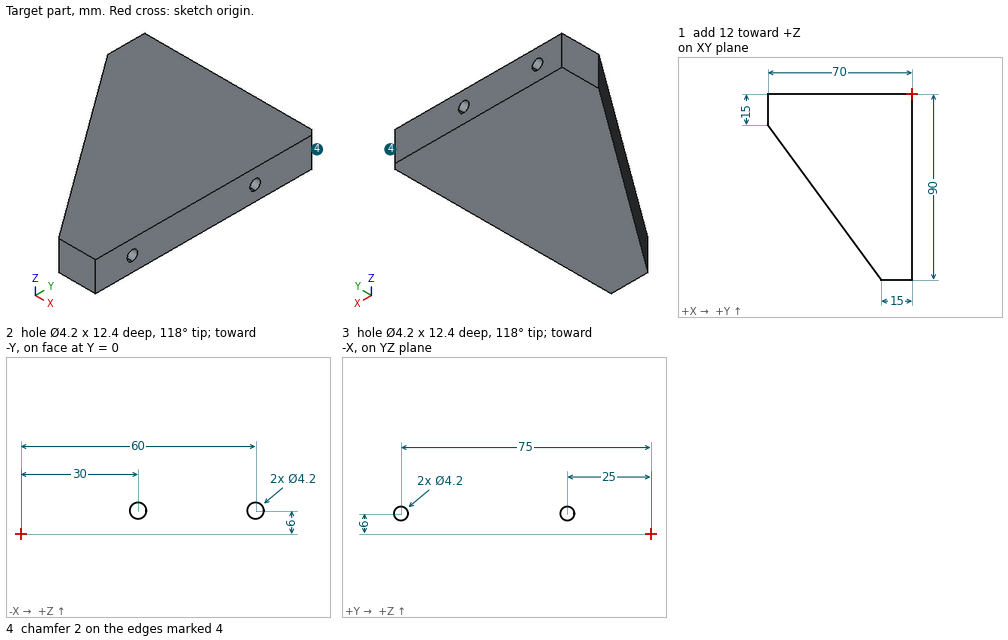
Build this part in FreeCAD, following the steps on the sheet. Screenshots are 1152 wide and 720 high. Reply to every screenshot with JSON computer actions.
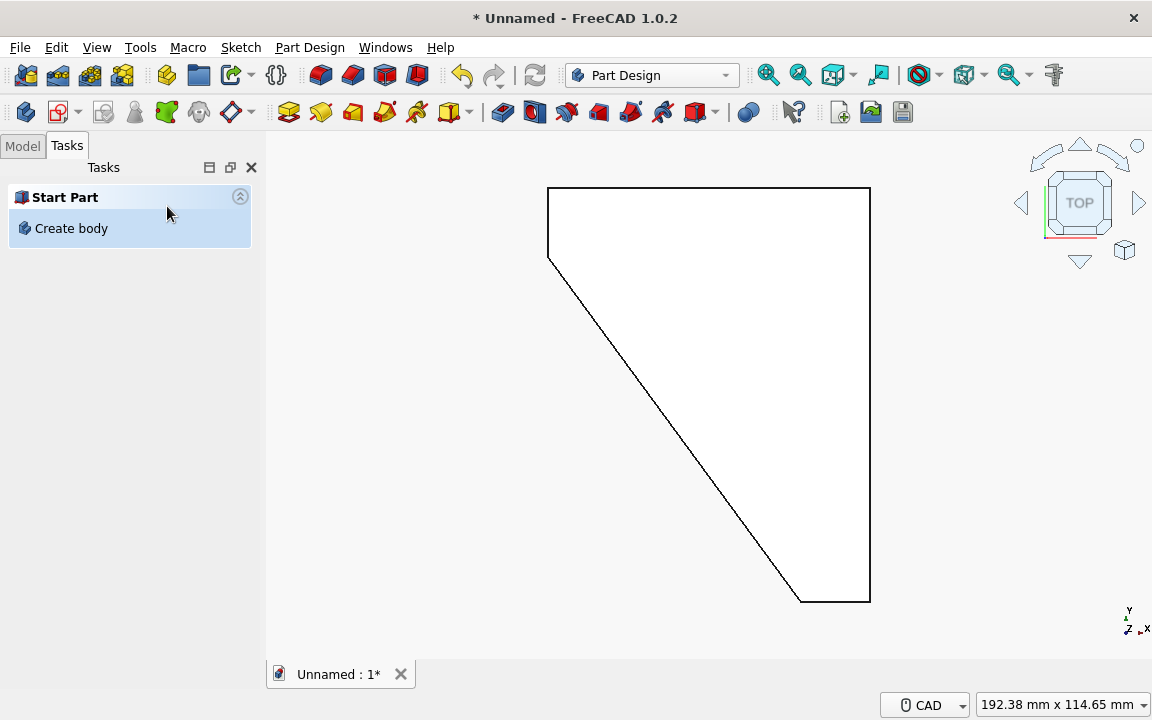
{"action": "key", "text": "1"}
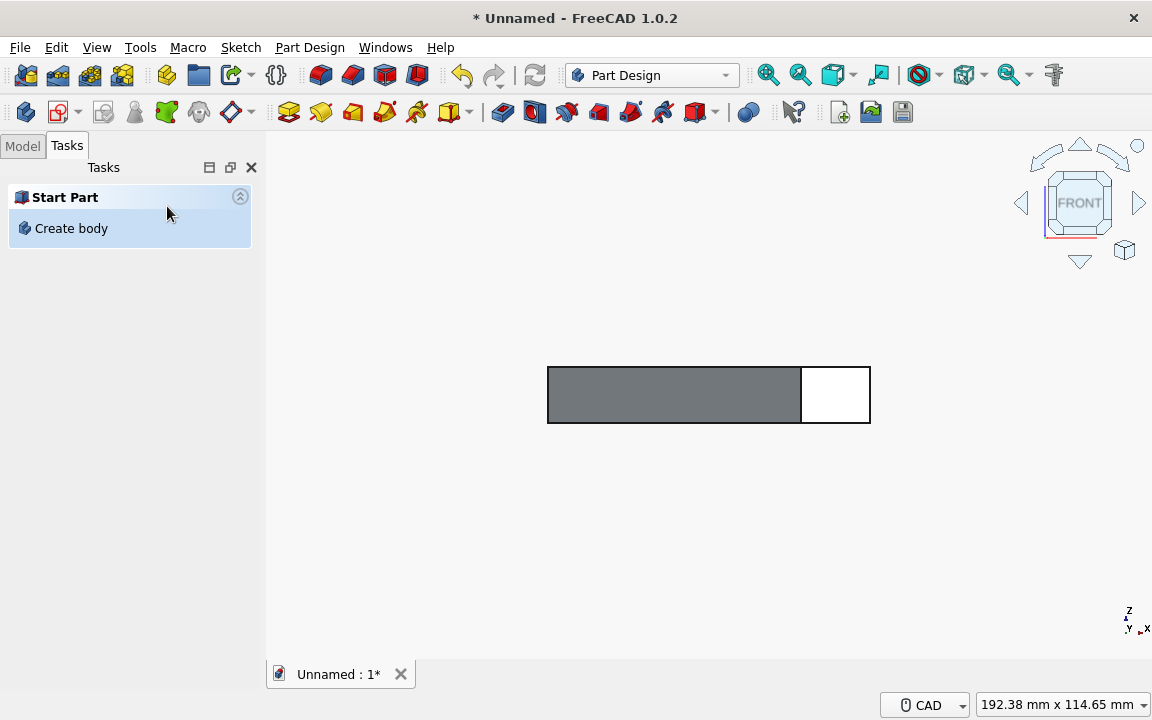
{"action": "left_click", "coordinate": [770, 76]}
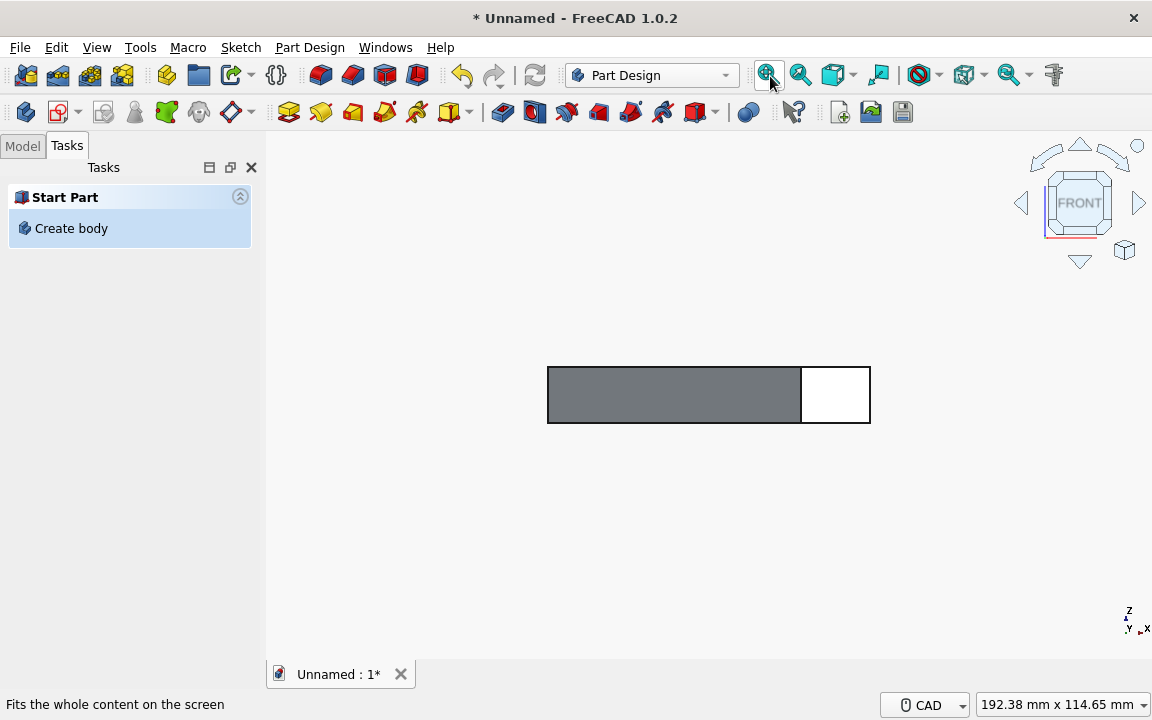
{"action": "key", "text": "3"}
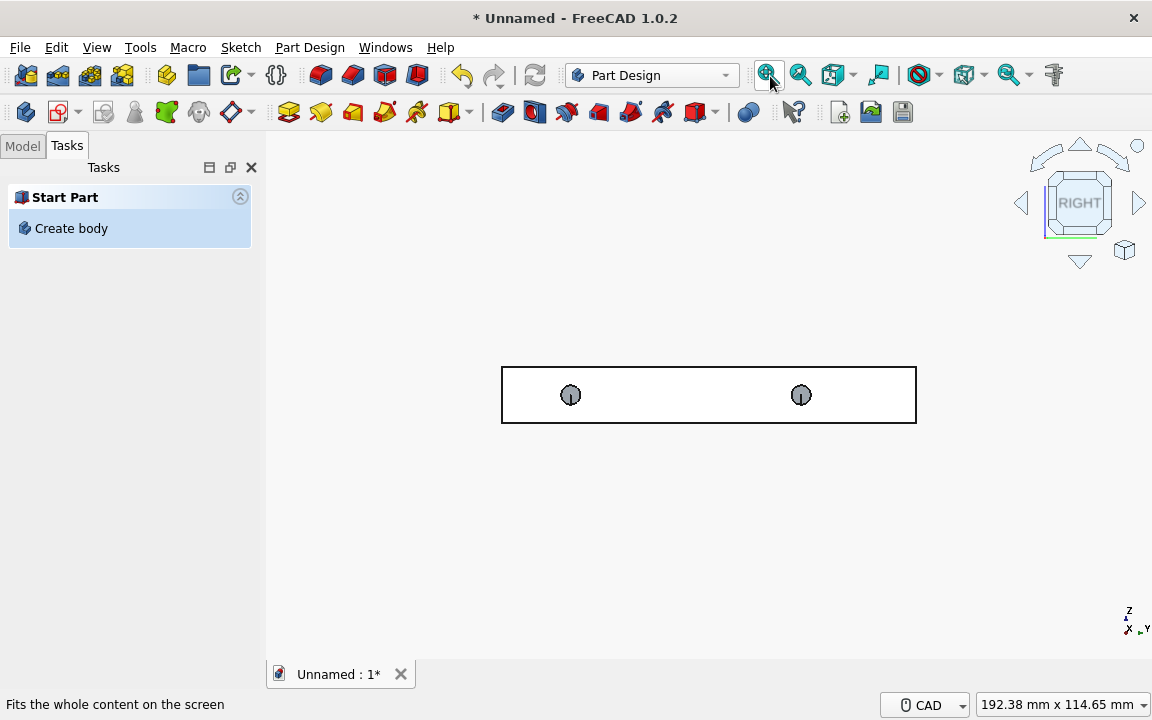
{"action": "left_click", "coordinate": [916, 394]}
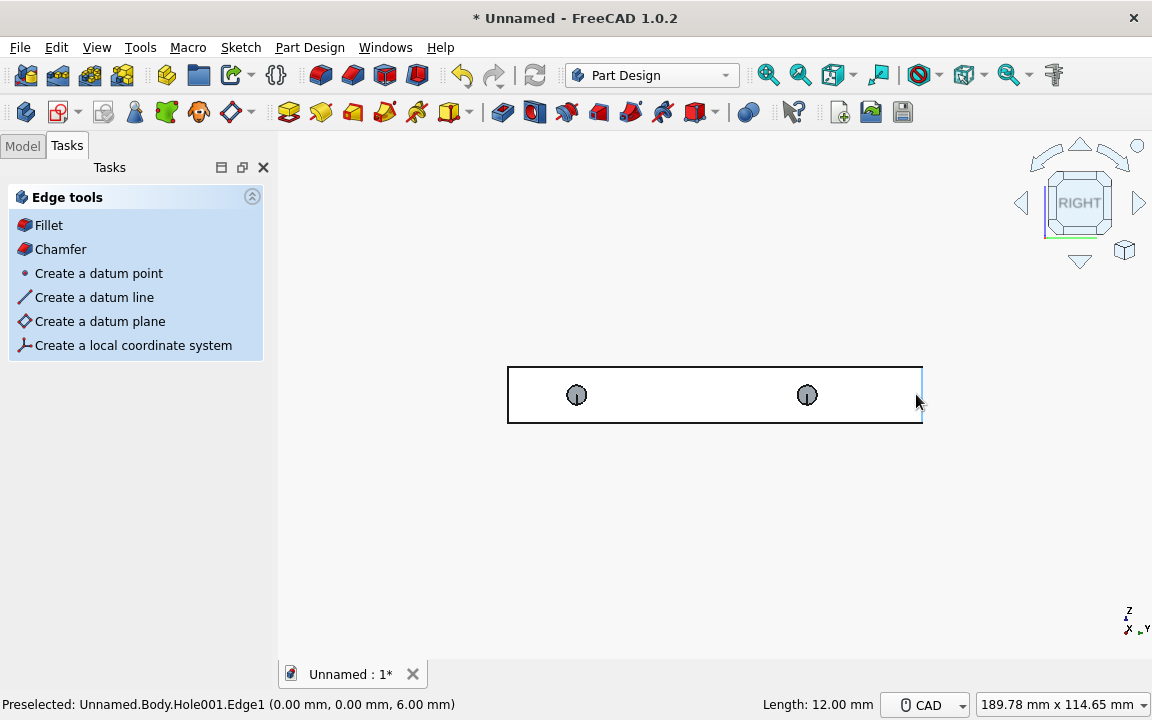
{"action": "left_click", "coordinate": [354, 76]}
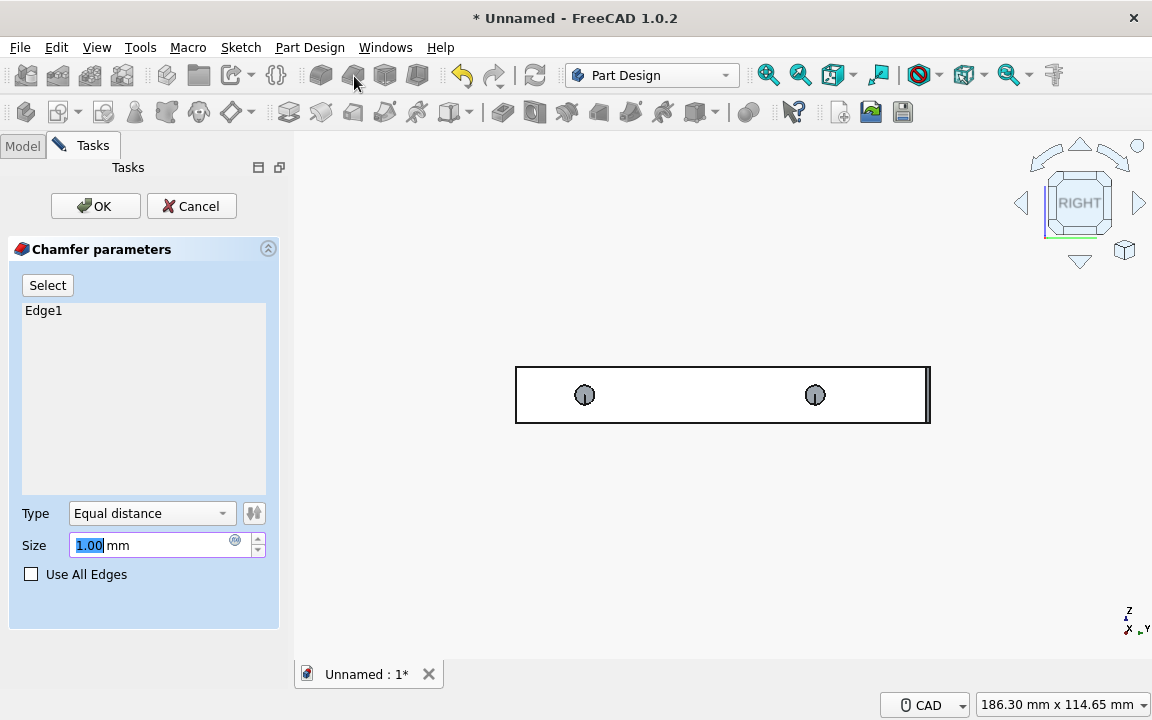
{"action": "type", "text": "2"}
{"action": "key", "text": "Tab"}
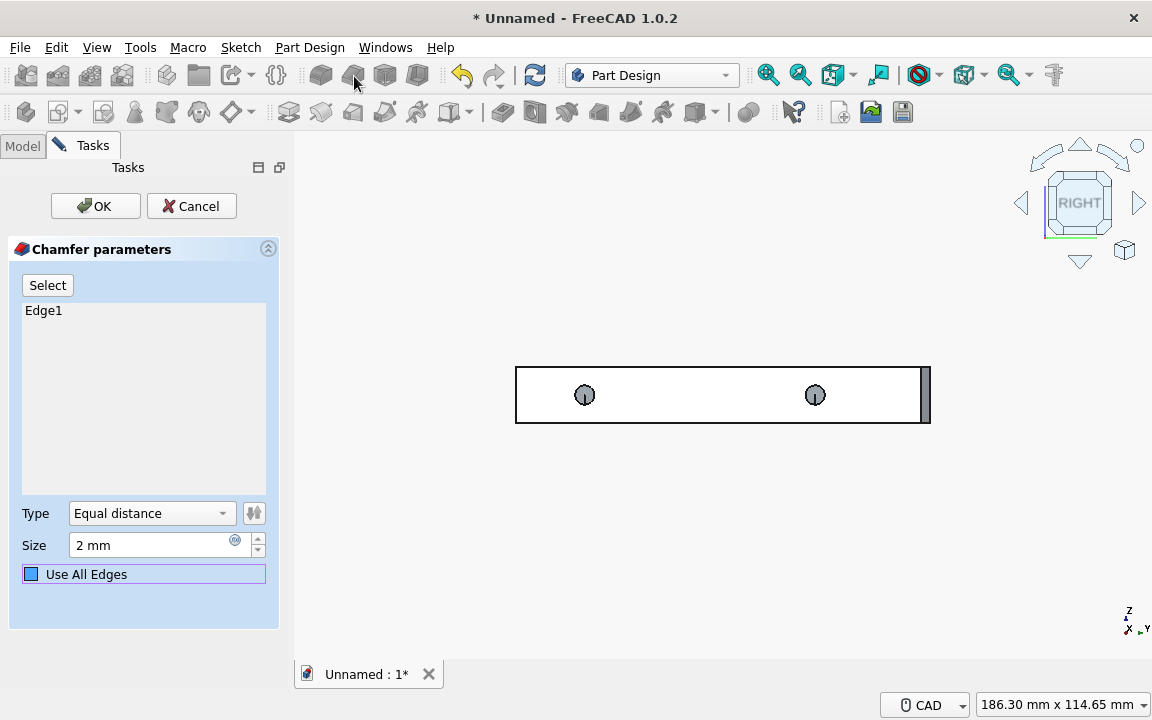
{"action": "left_click", "coordinate": [96, 206]}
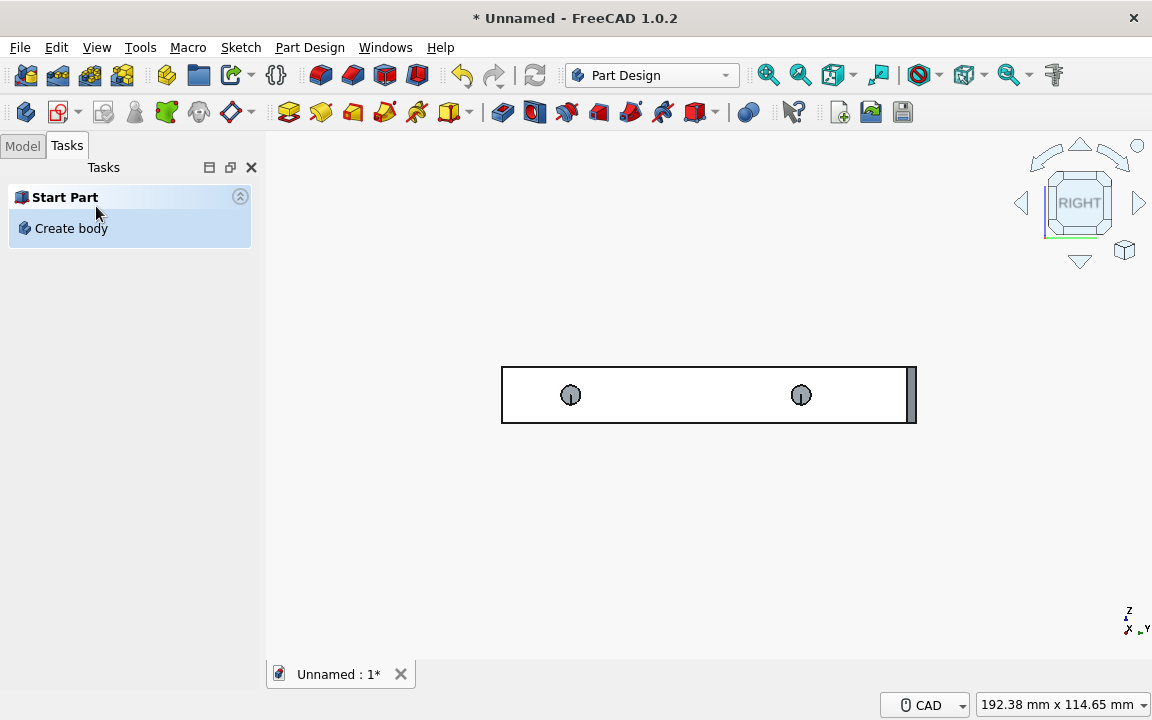
{"action": "key", "text": "0"}